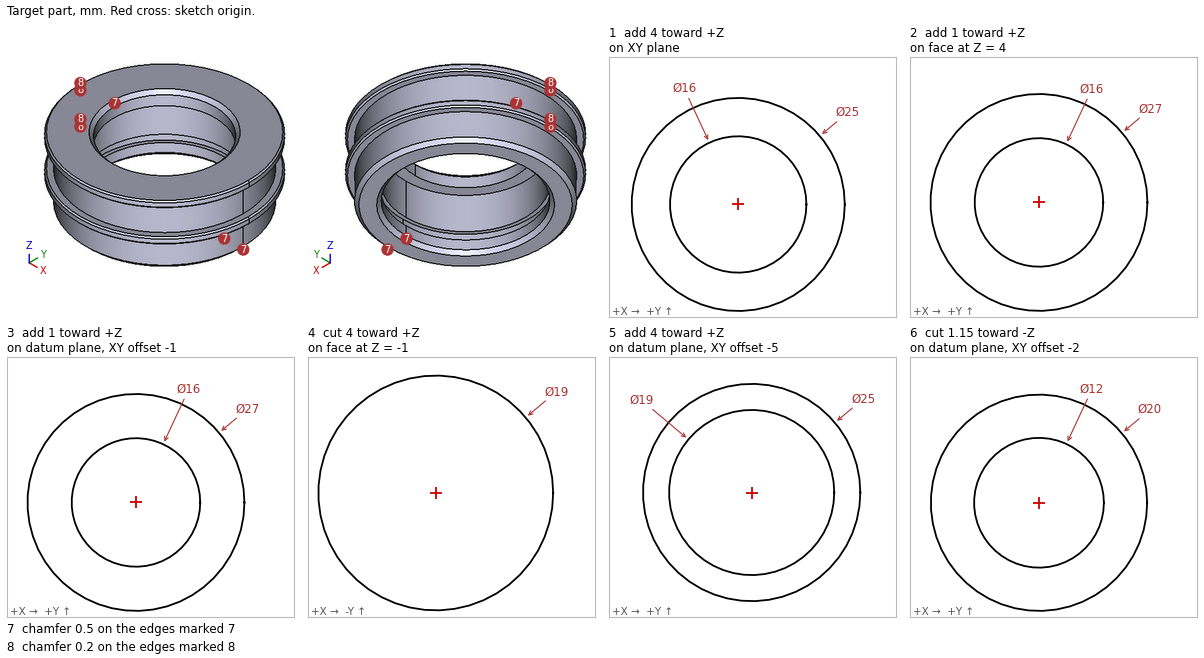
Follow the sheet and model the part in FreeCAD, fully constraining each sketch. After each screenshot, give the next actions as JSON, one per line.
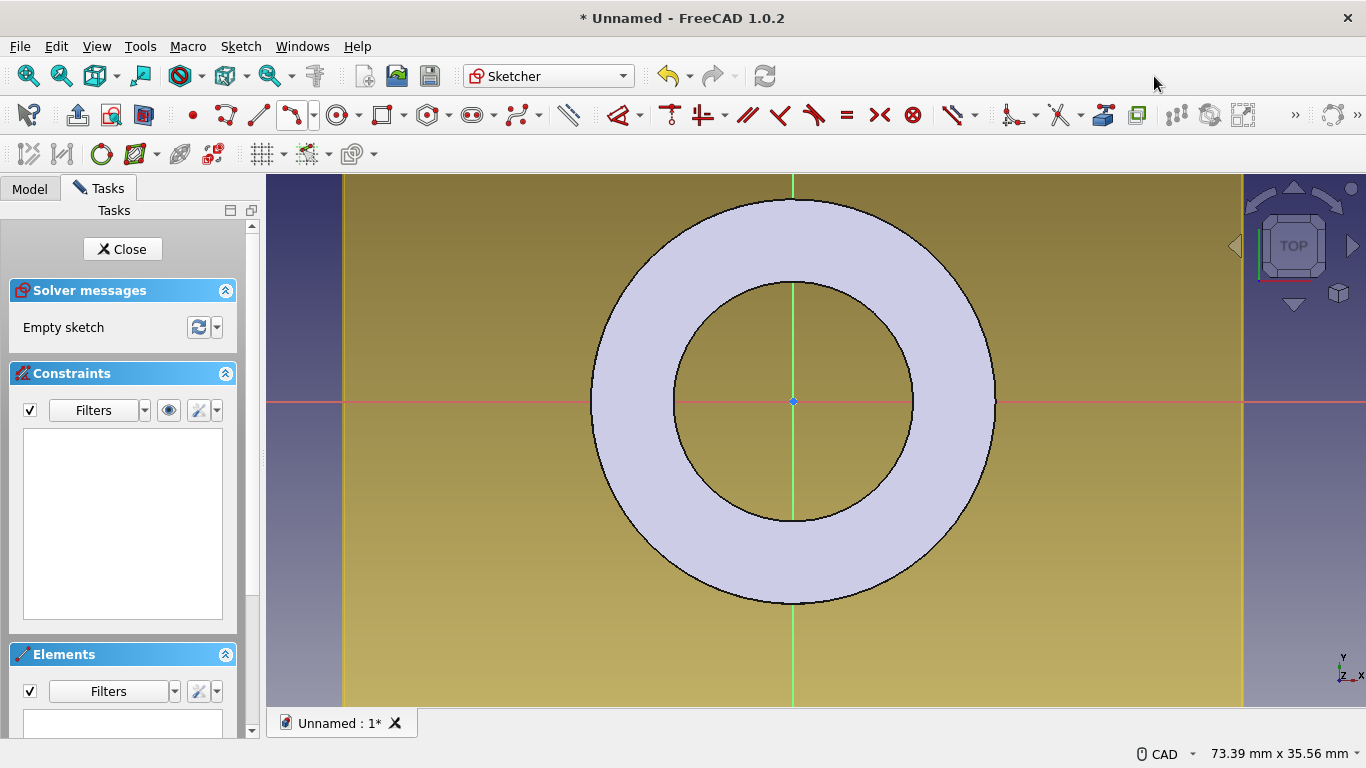
{"action": "left_click", "coordinate": [144, 116]}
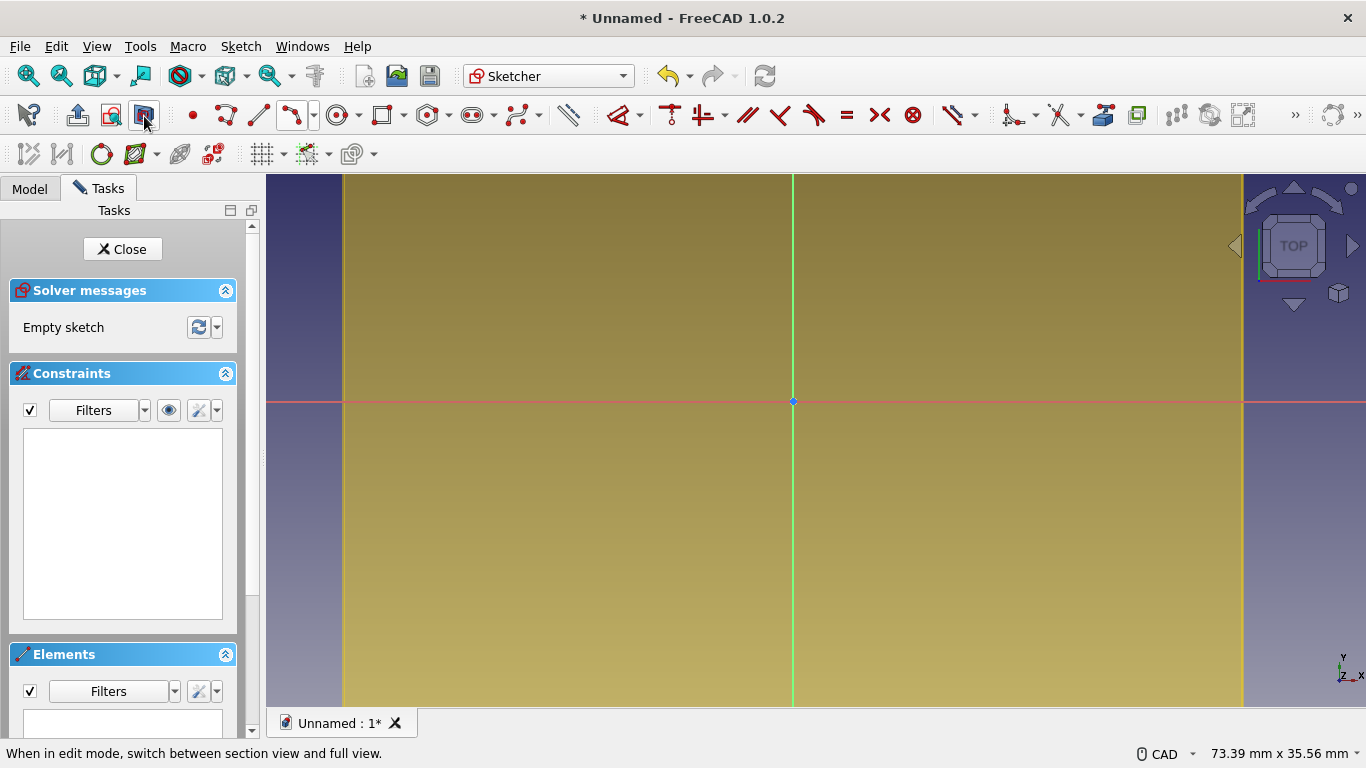
{"action": "scroll", "coordinate": [541, 616], "scroll_direction": "down", "scroll_amount": 1}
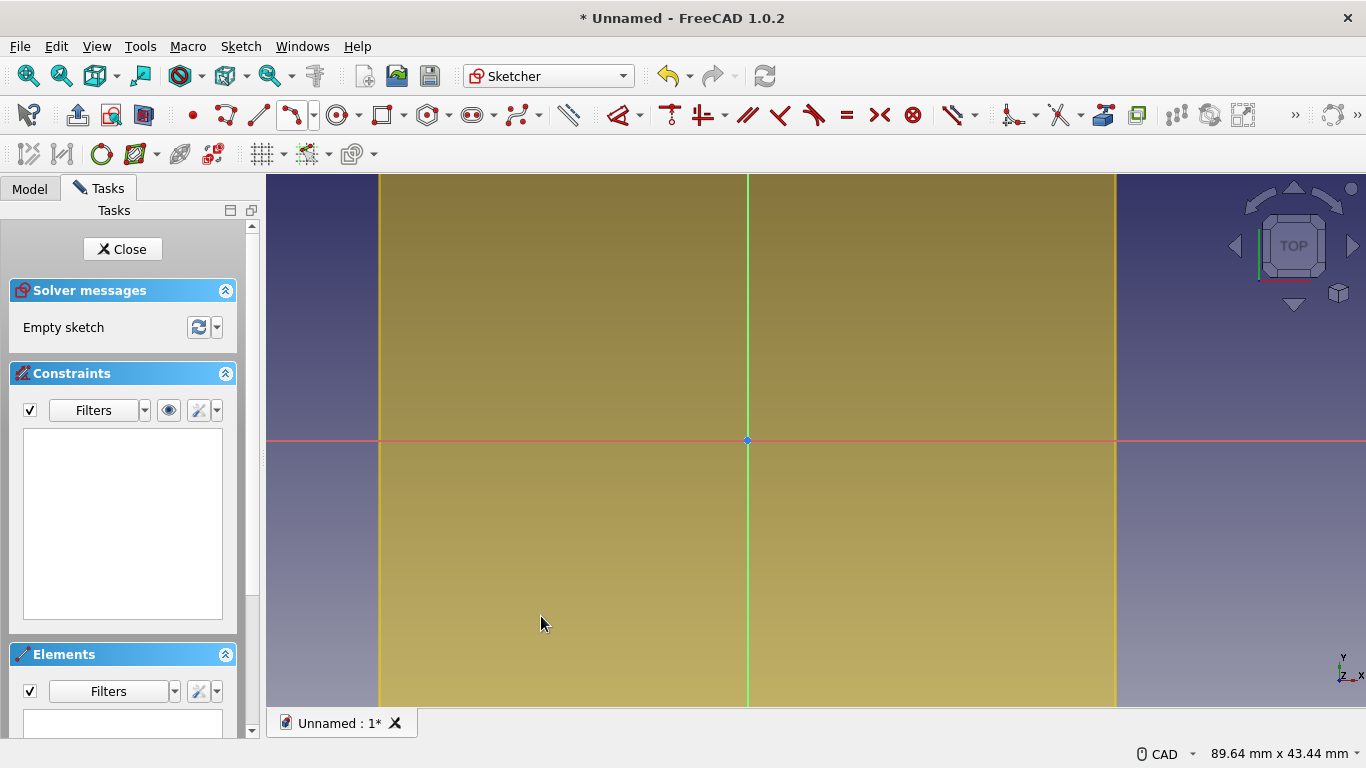
{"action": "left_click", "coordinate": [336, 116]}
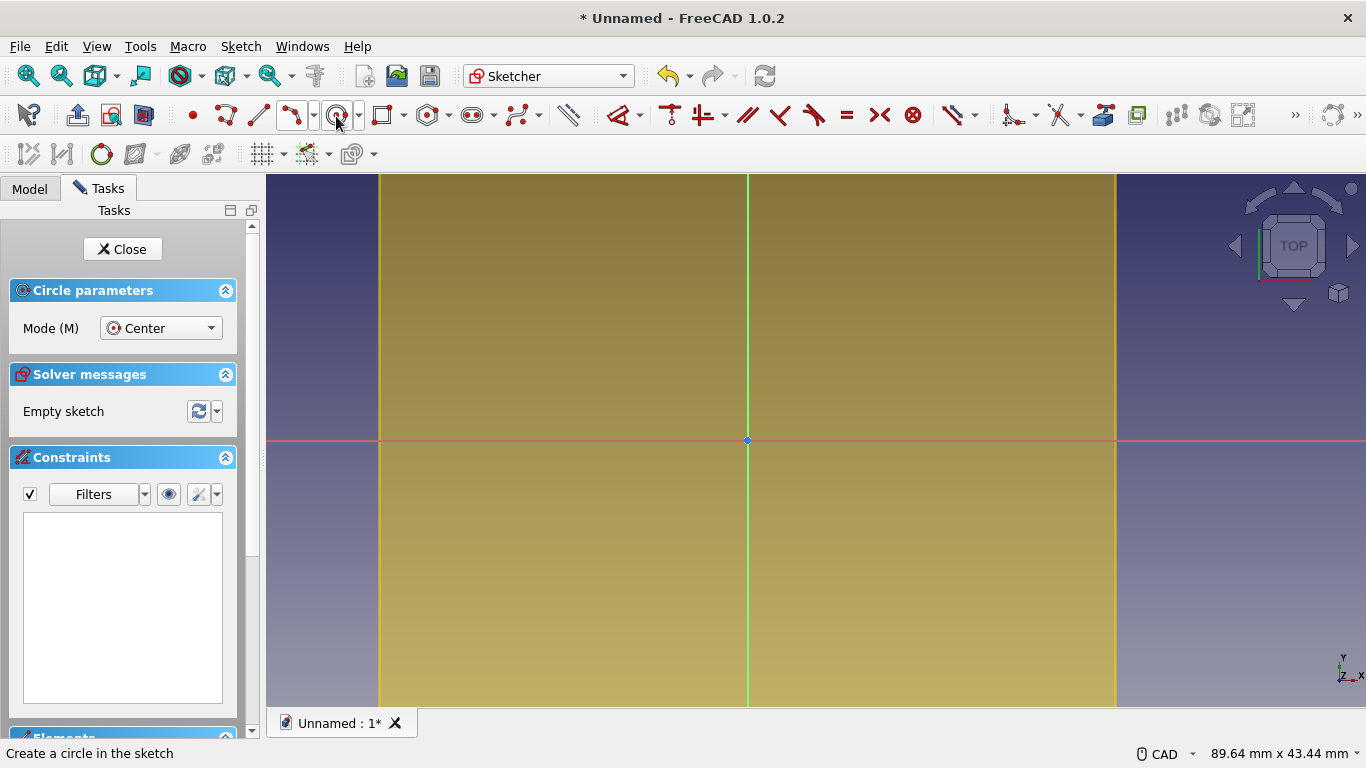
{"action": "left_click", "coordinate": [748, 441]}
{"action": "left_click", "coordinate": [856, 332]}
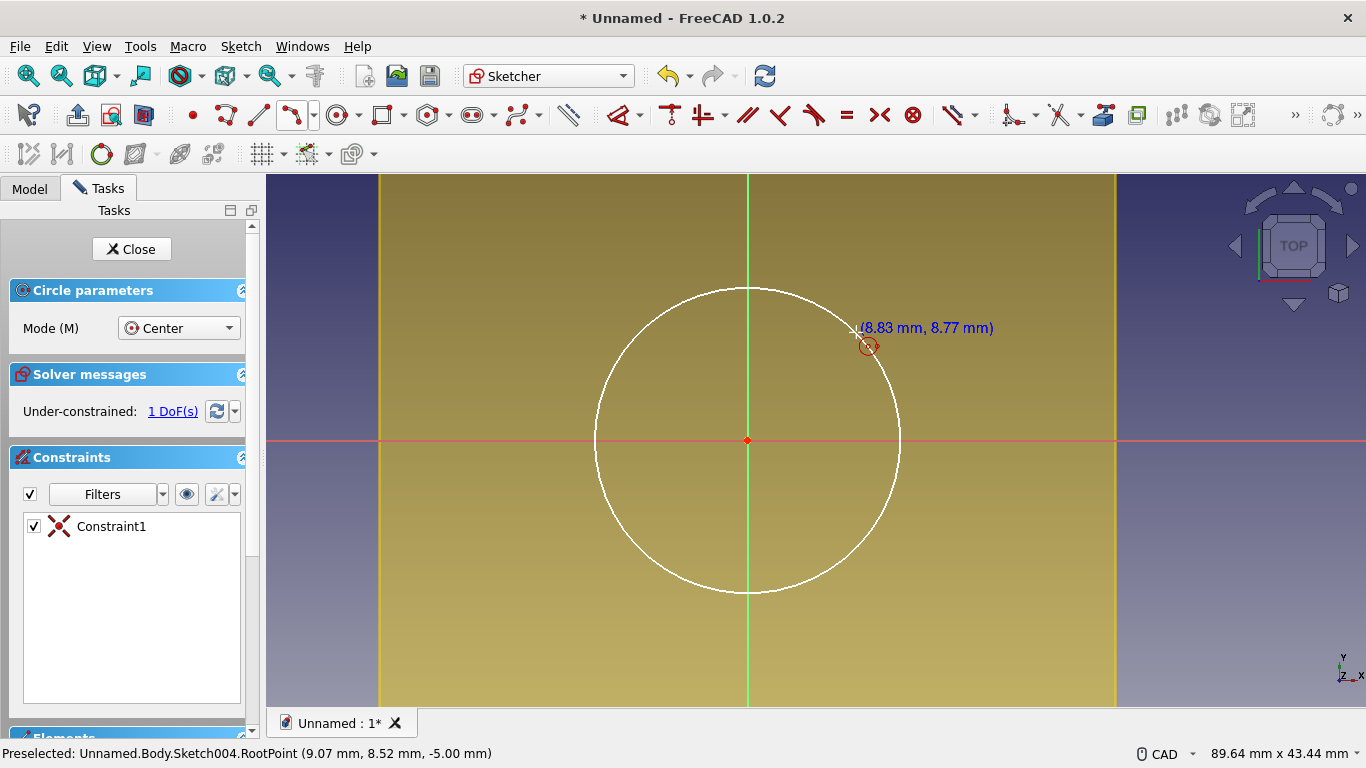
{"action": "left_click", "coordinate": [748, 441]}
{"action": "left_click", "coordinate": [830, 358]}
{"action": "key", "text": "Escape"}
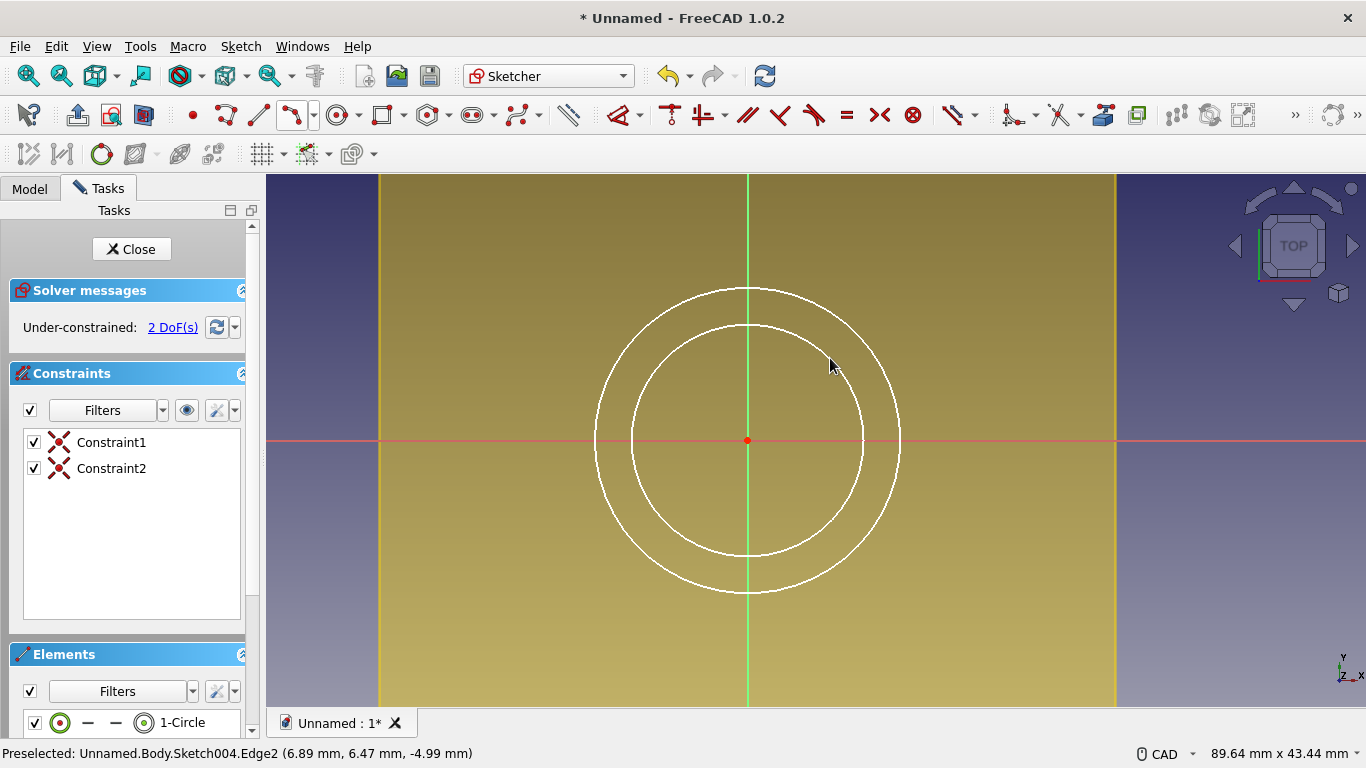
{"action": "left_click", "coordinate": [618, 116]}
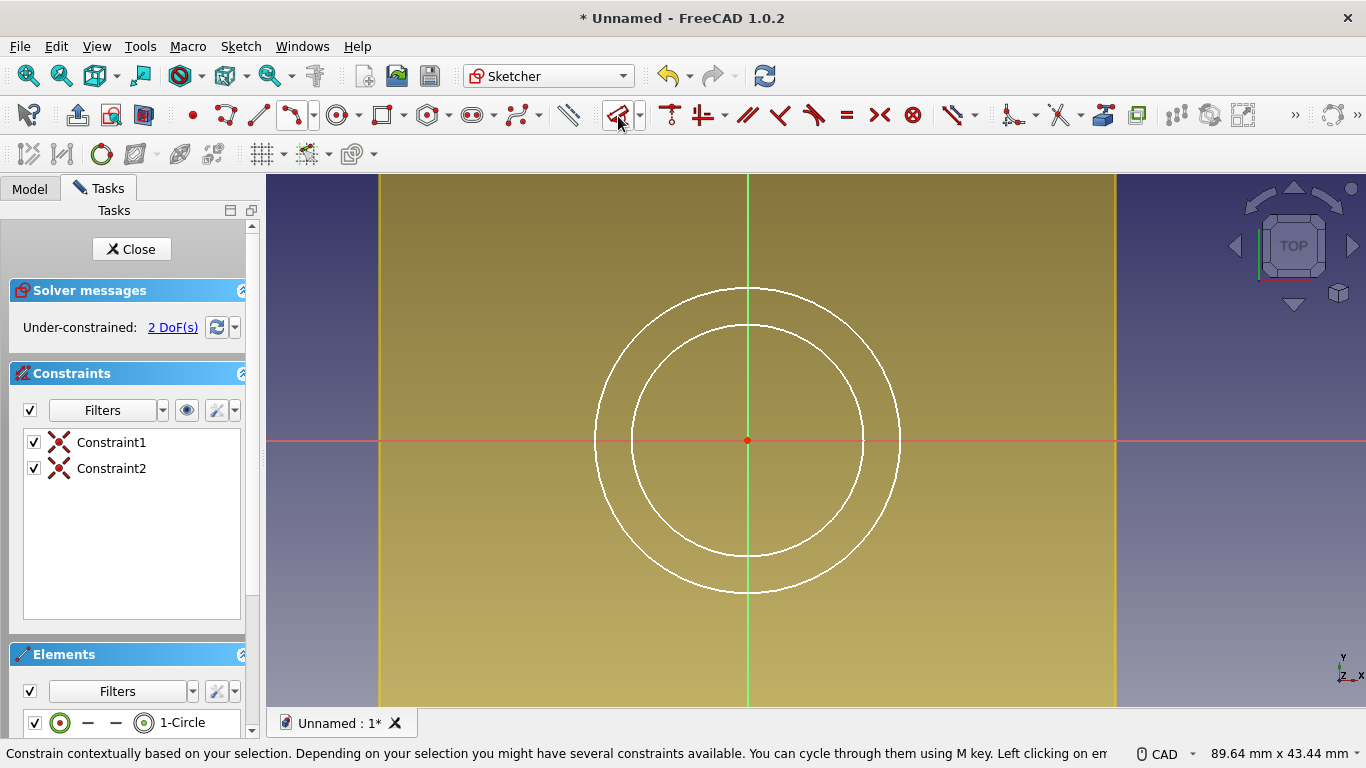
{"action": "left_click", "coordinate": [855, 332]}
{"action": "left_click", "coordinate": [878, 309]}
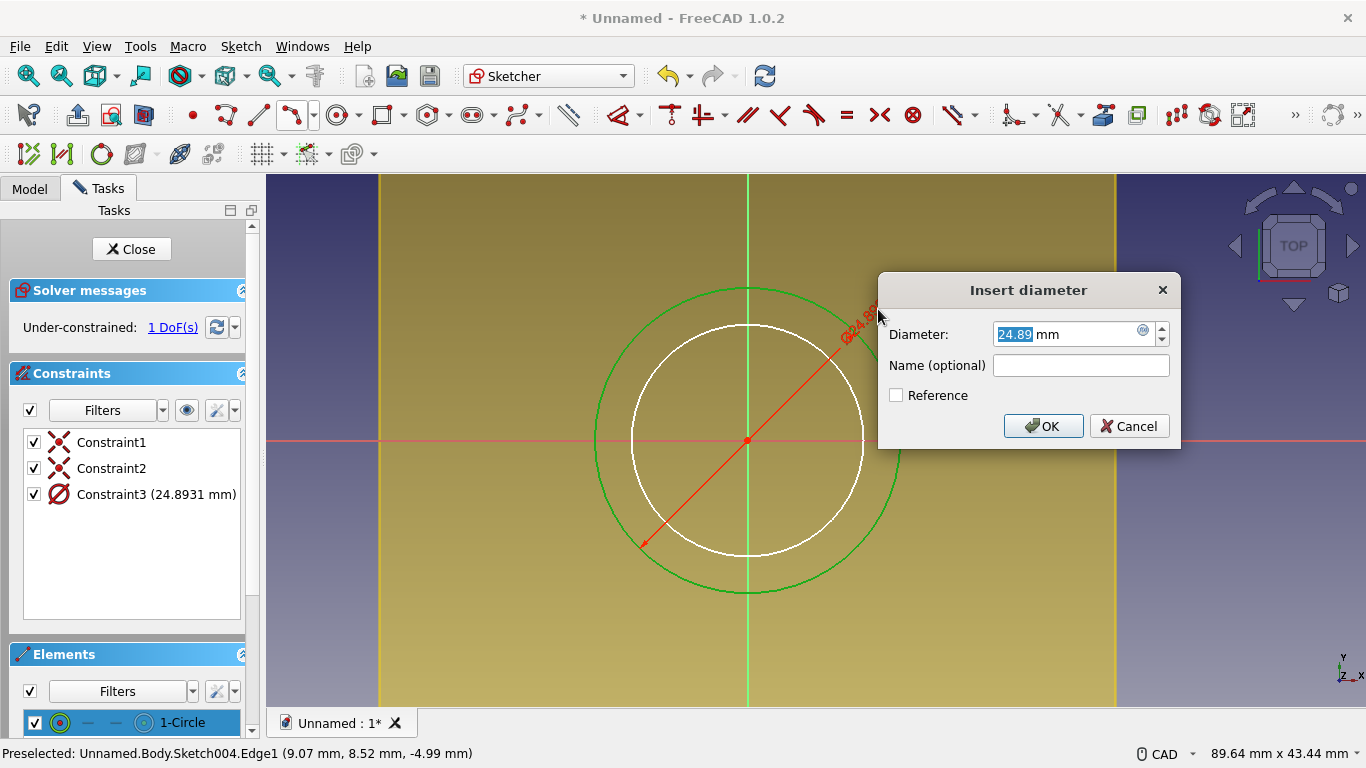
{"action": "type", "text": "25"}
{"action": "key", "text": "Return"}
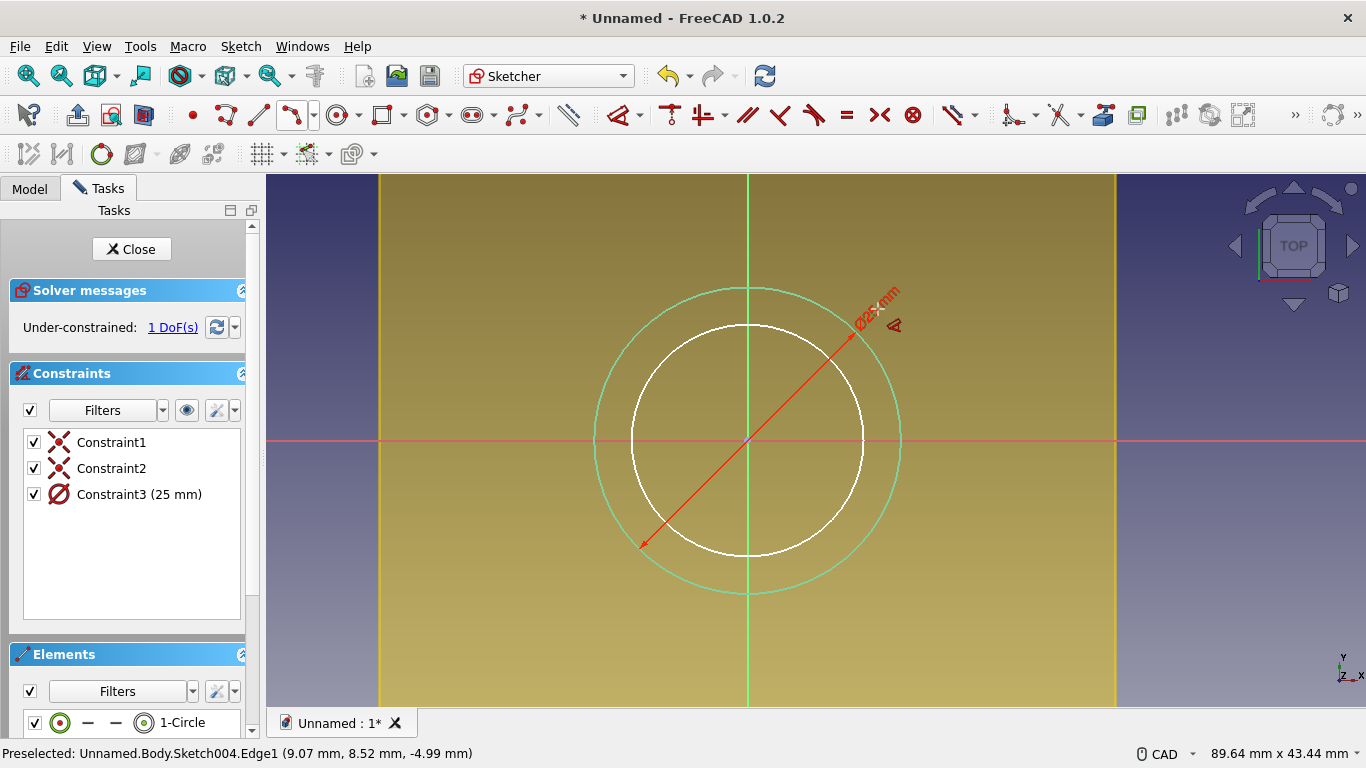
{"action": "left_click", "coordinate": [829, 358]}
{"action": "left_click", "coordinate": [911, 391]}